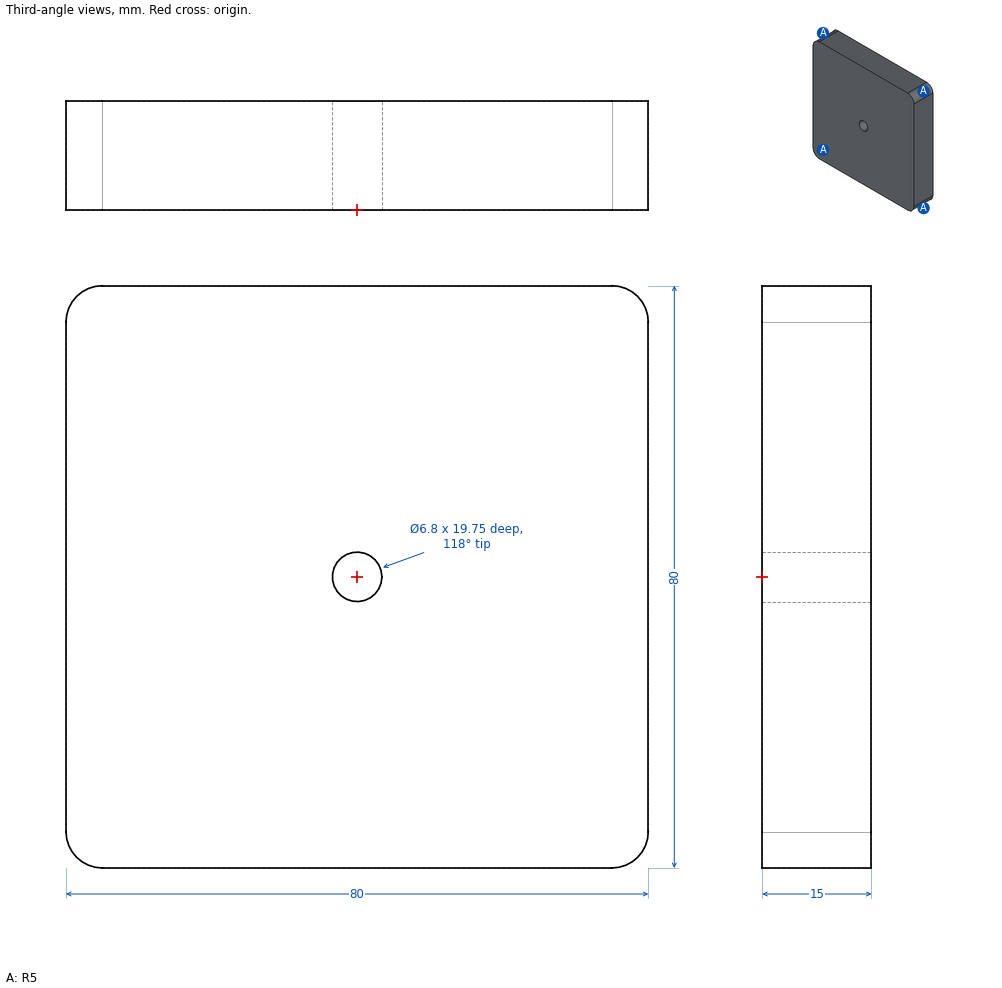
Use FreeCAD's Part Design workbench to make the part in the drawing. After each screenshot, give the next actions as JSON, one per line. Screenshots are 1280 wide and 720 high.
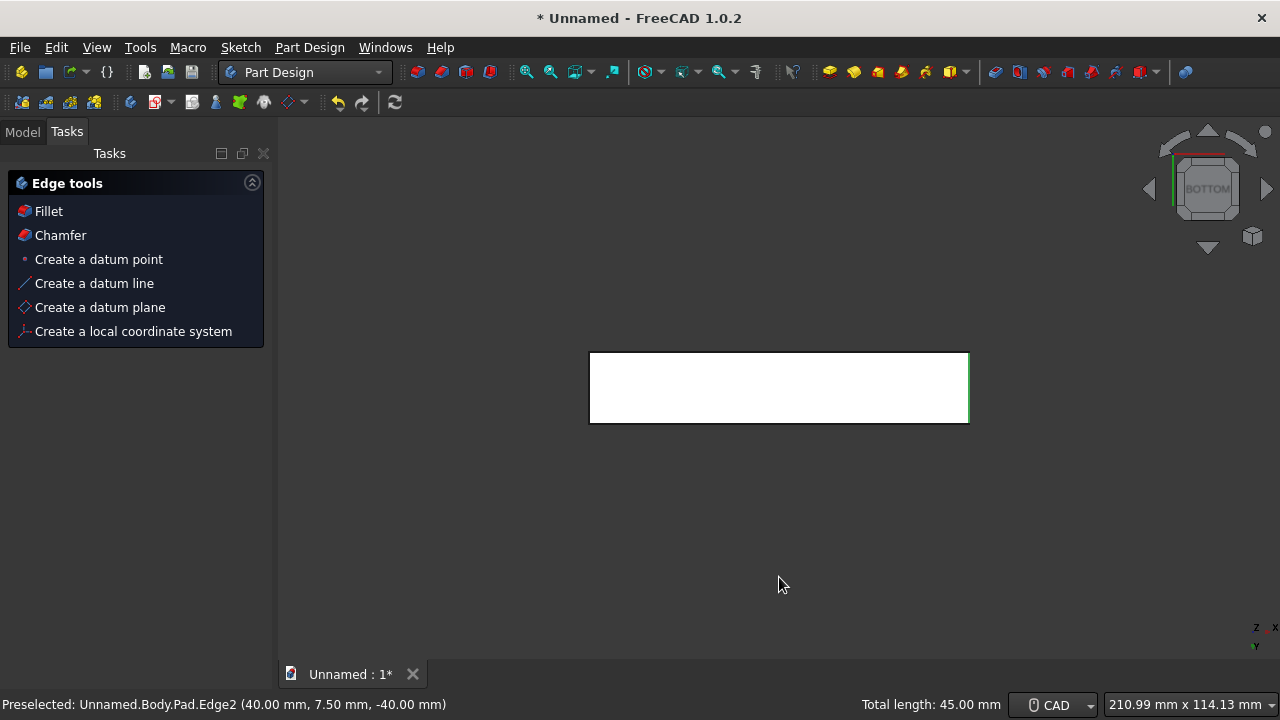
{"action": "key", "text": "v f"}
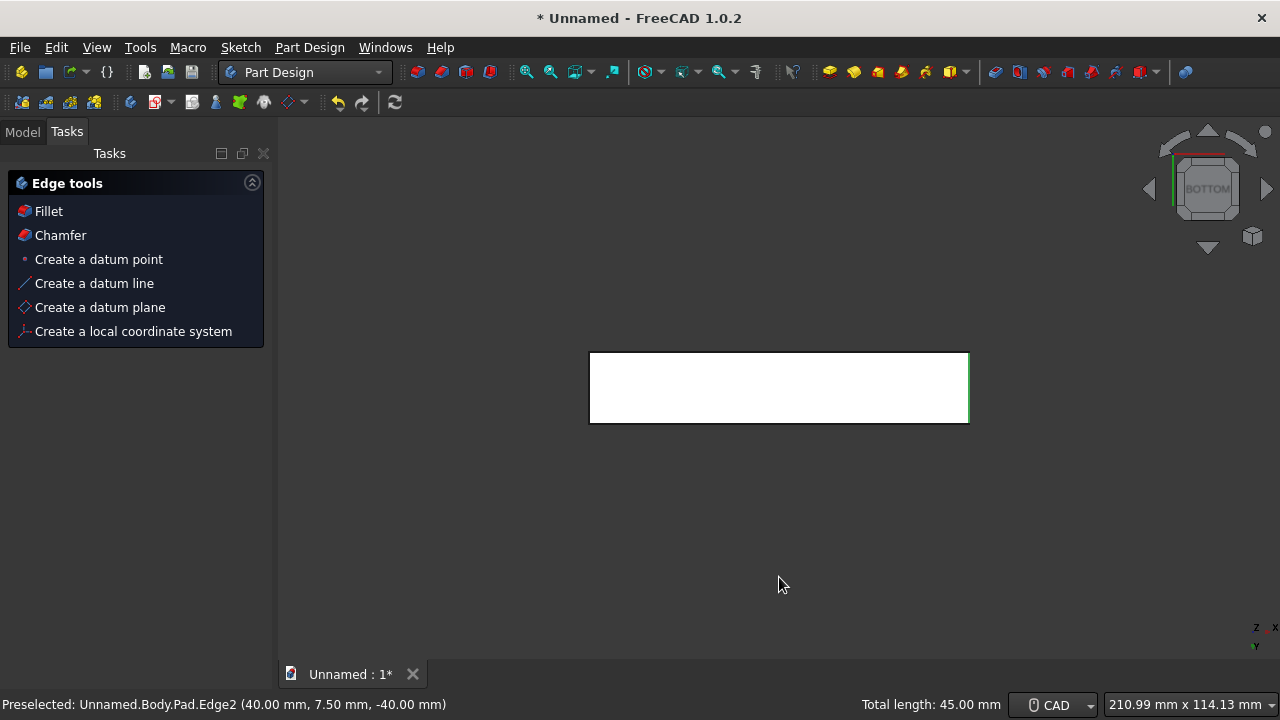
{"action": "left_click", "coordinate": [589, 387], "text": "ctrl"}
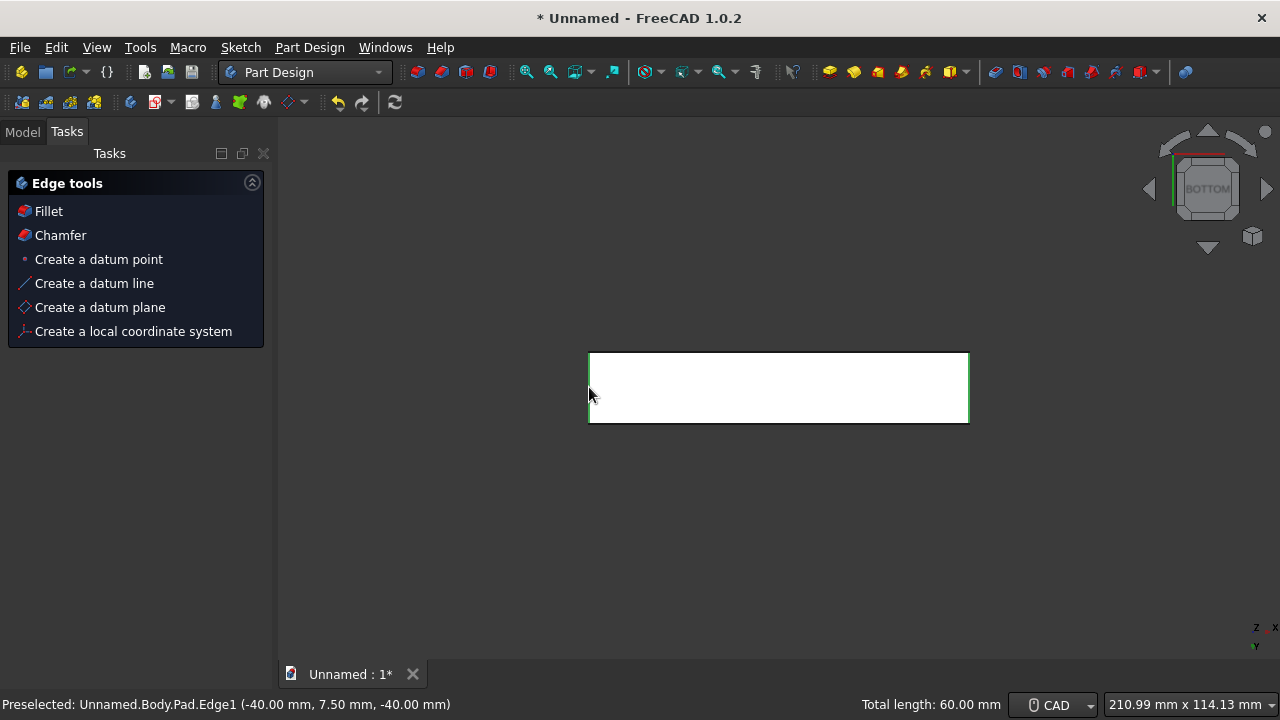
{"action": "left_click", "coordinate": [418, 72]}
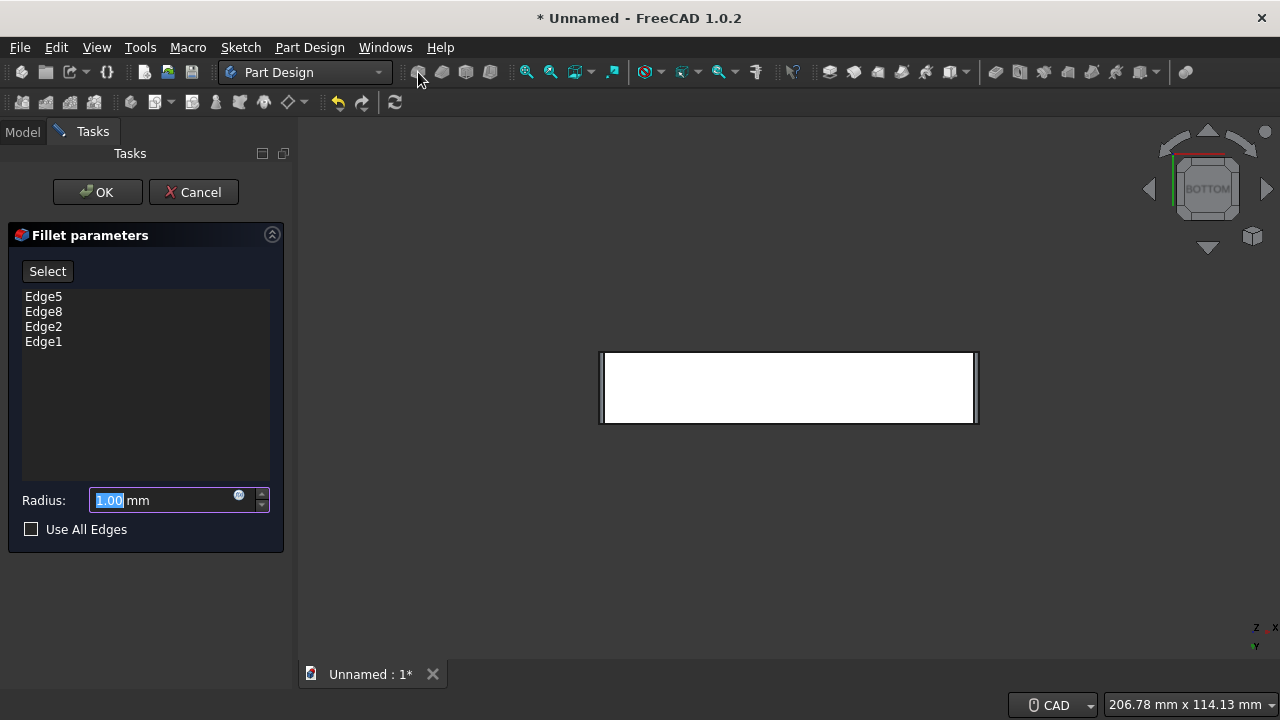
{"action": "type", "text": "5"}
{"action": "key", "text": "Tab"}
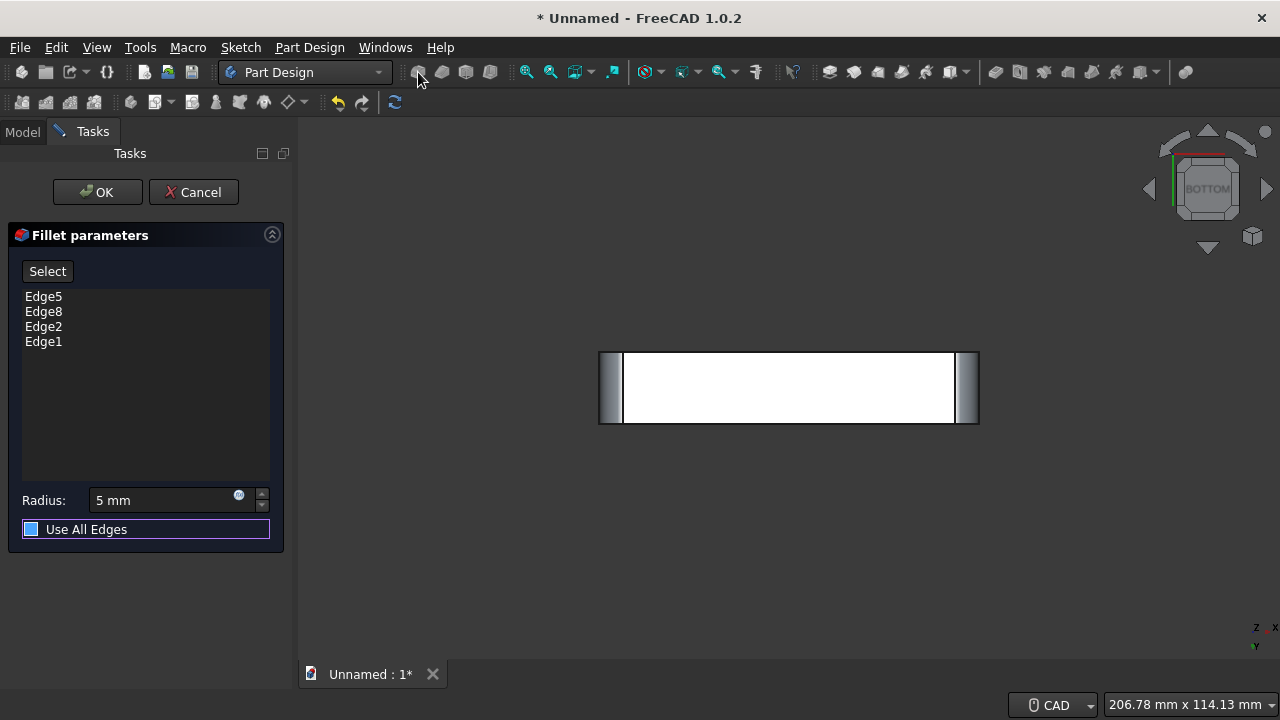
{"action": "left_click", "coordinate": [98, 192]}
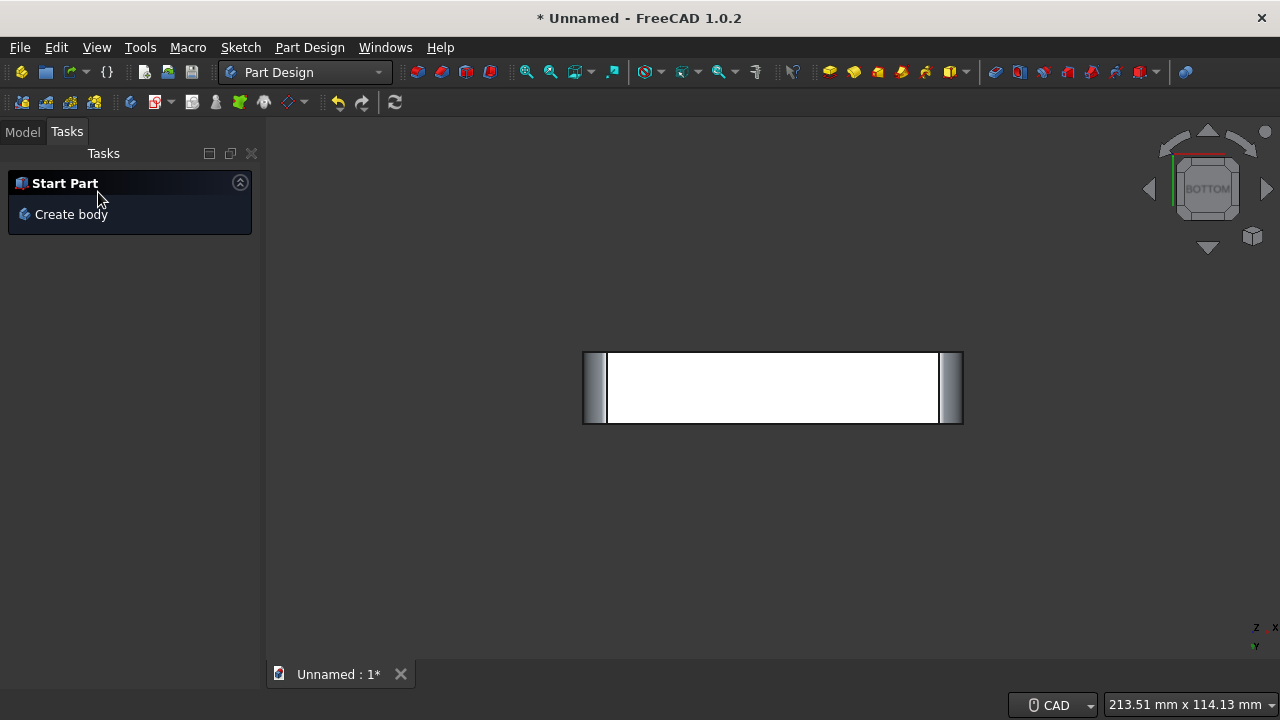
{"action": "left_click", "coordinate": [528, 72]}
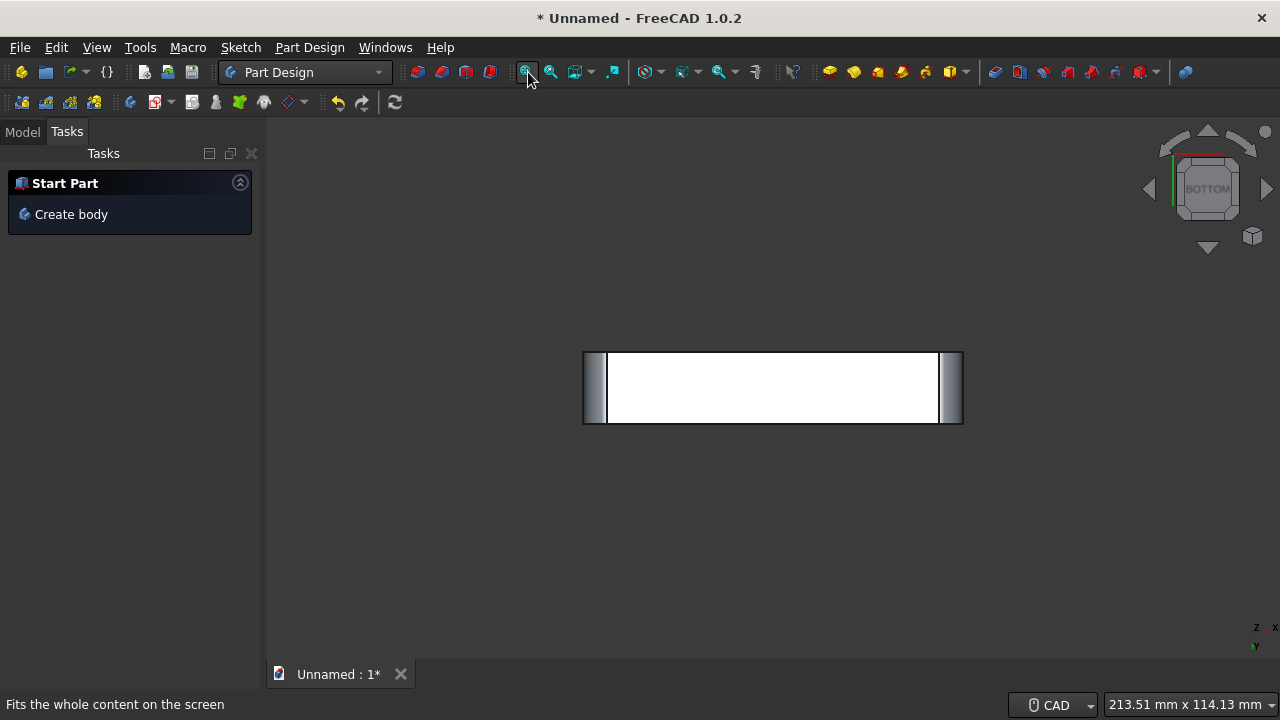
{"action": "key", "text": "0"}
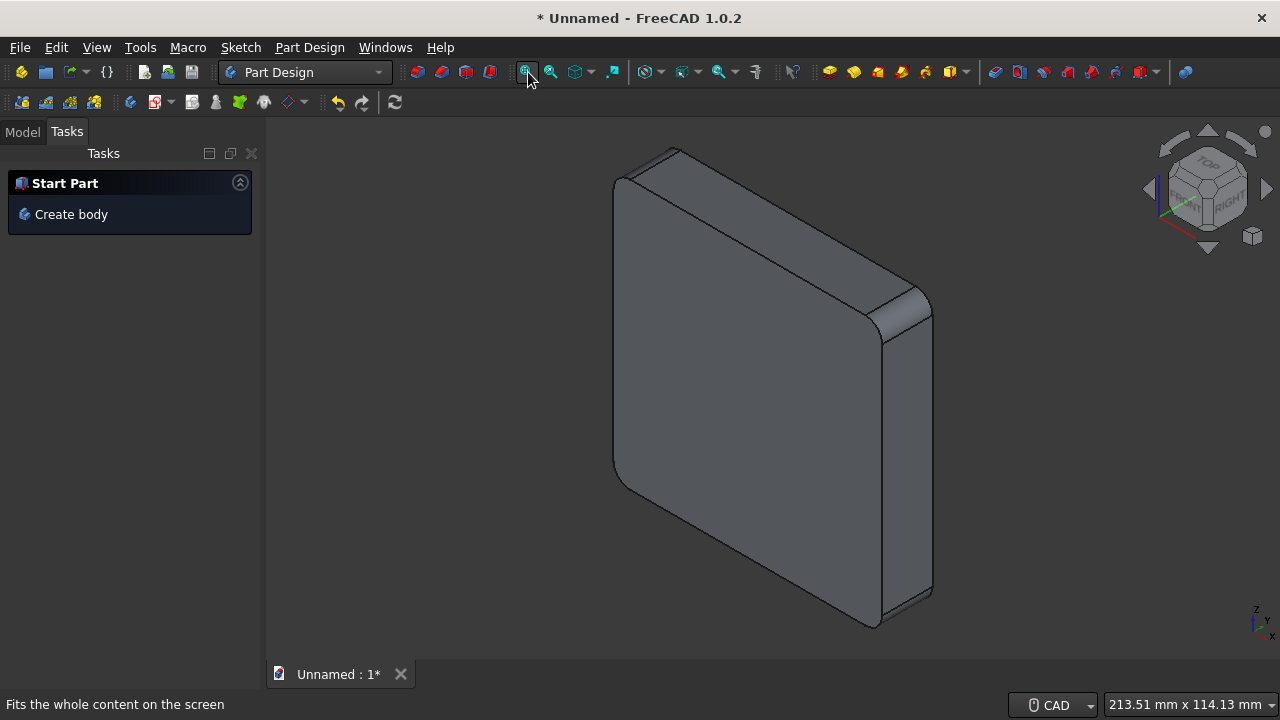
{"action": "left_click", "coordinate": [748, 402]}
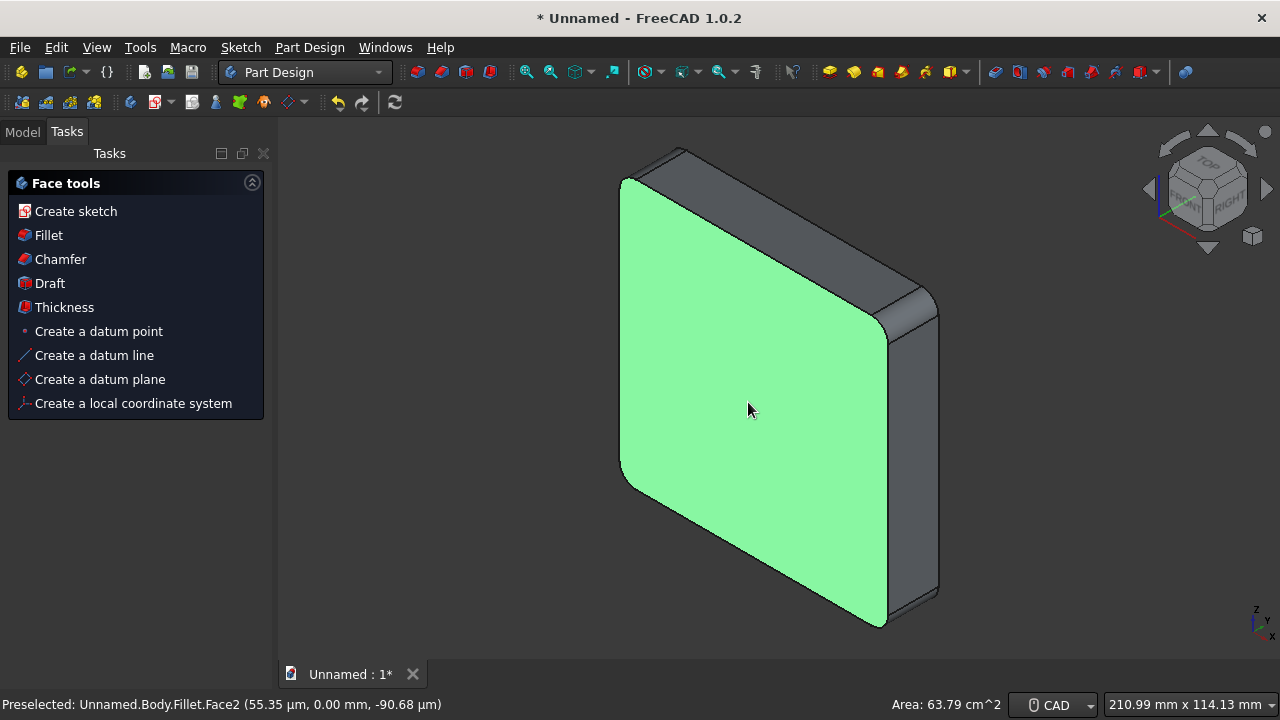
{"action": "left_click", "coordinate": [156, 102]}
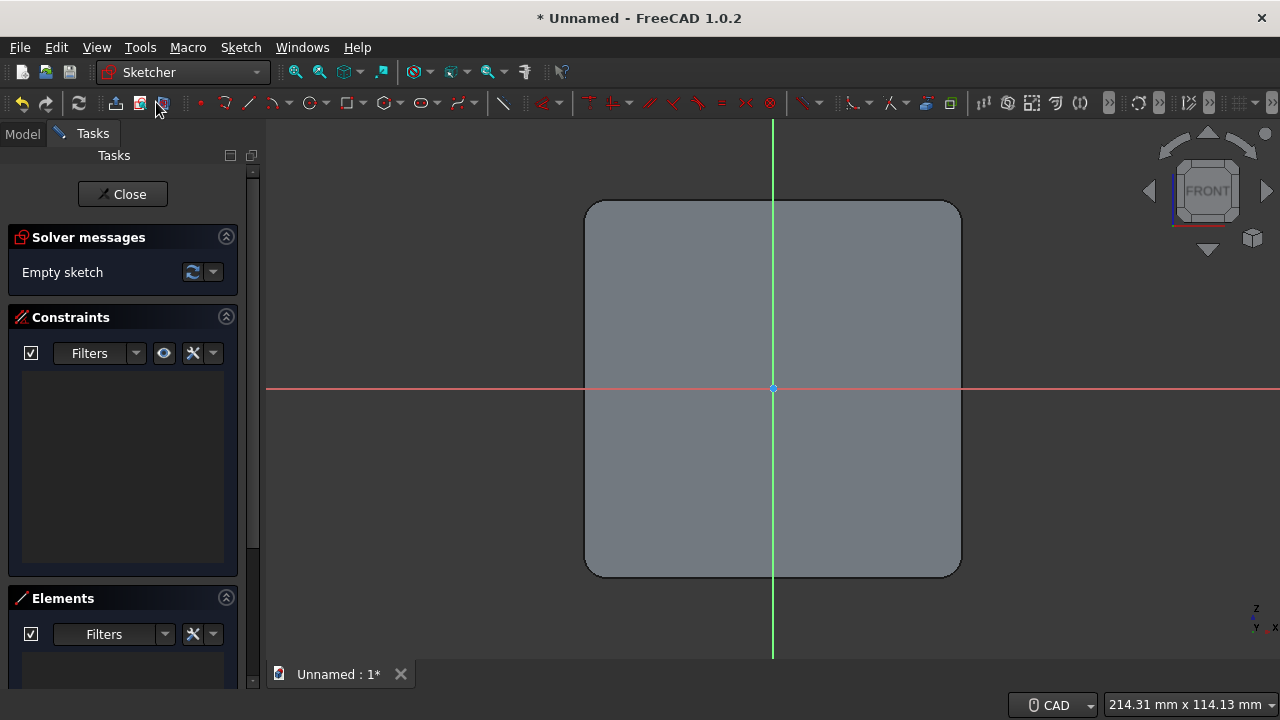
{"action": "scroll", "coordinate": [780, 389], "scroll_direction": "up", "scroll_amount": 12}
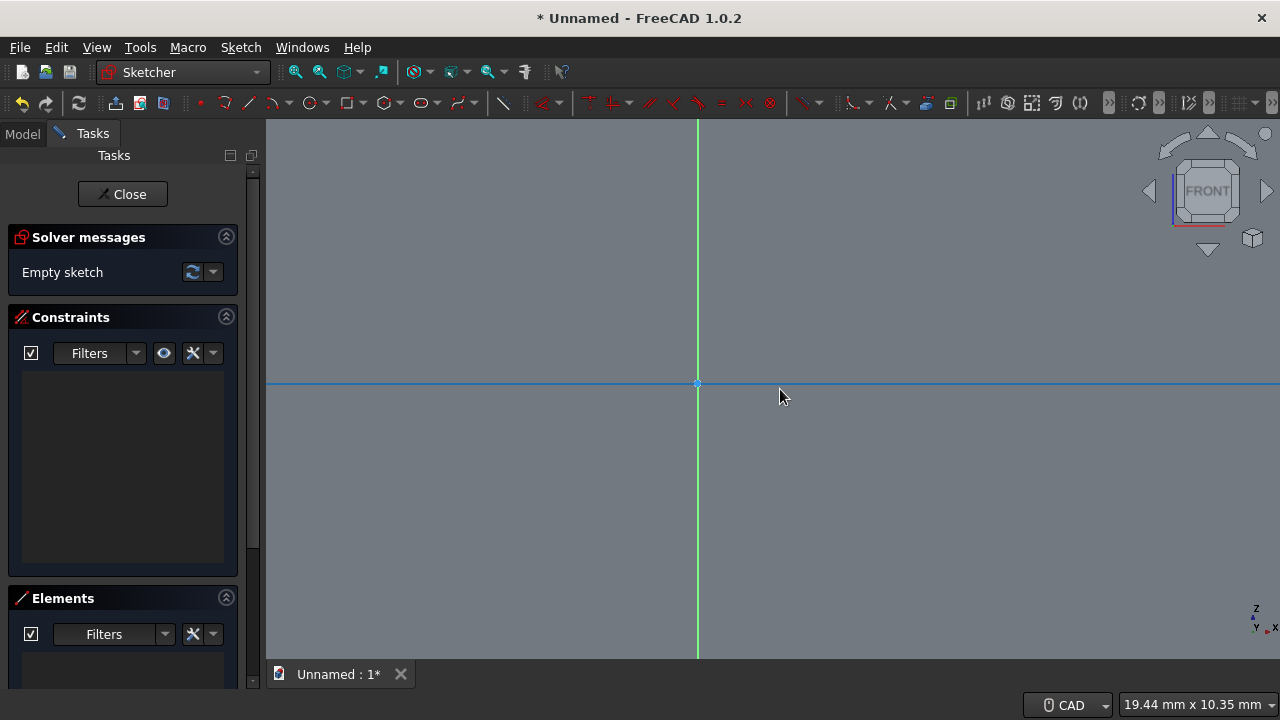
{"action": "key", "text": "g c"}